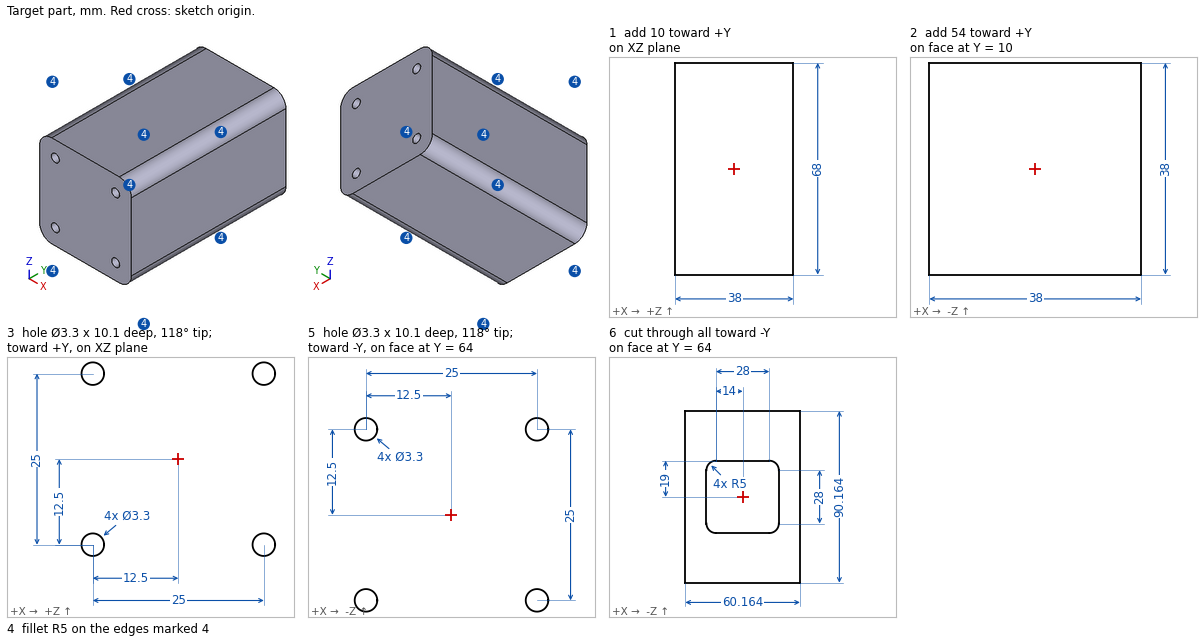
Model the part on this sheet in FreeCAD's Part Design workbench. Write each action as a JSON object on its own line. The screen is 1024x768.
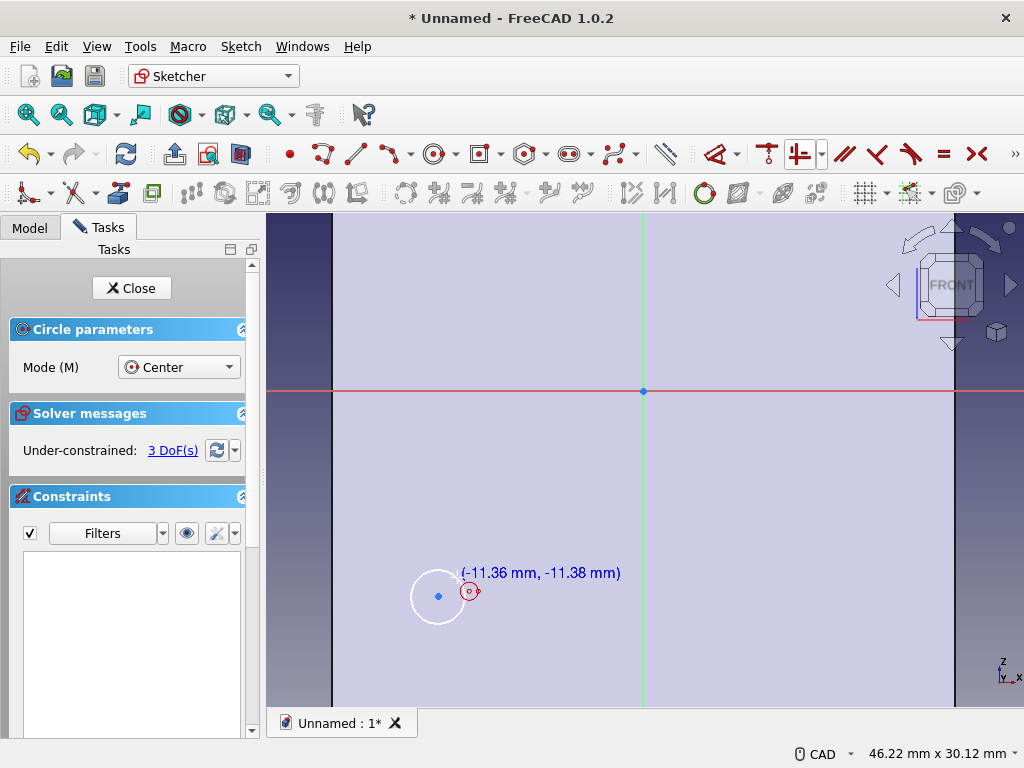
{"action": "left_click", "coordinate": [848, 596]}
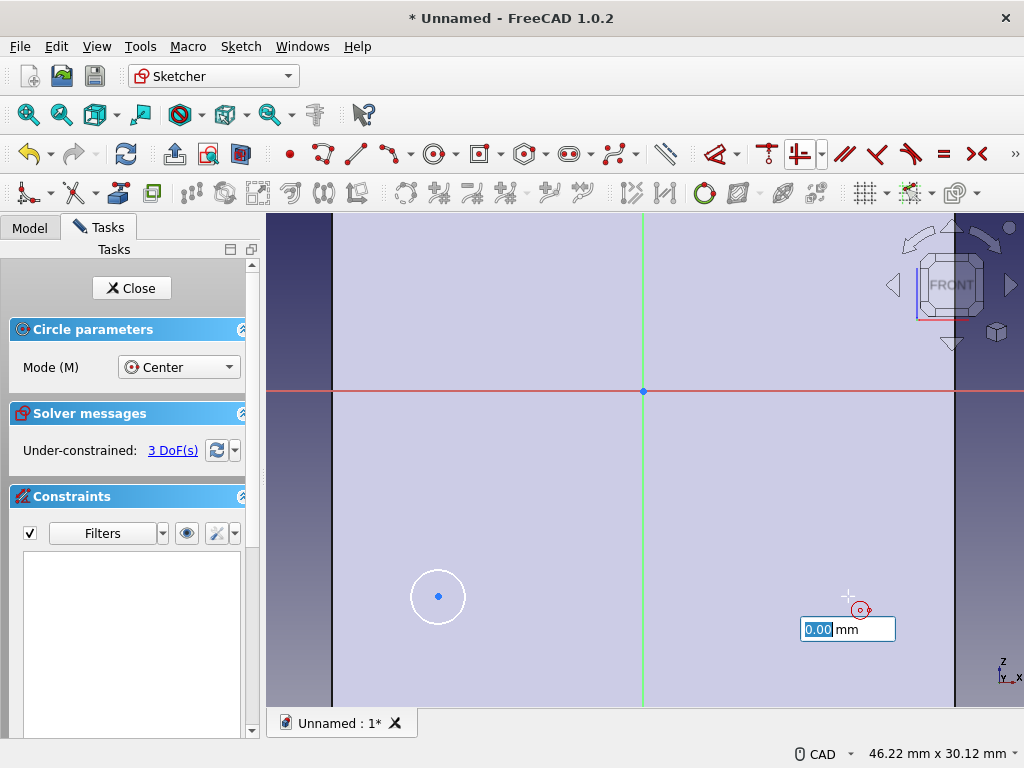
{"action": "scroll", "coordinate": [441, 600], "scroll_direction": "down", "scroll_amount": 2}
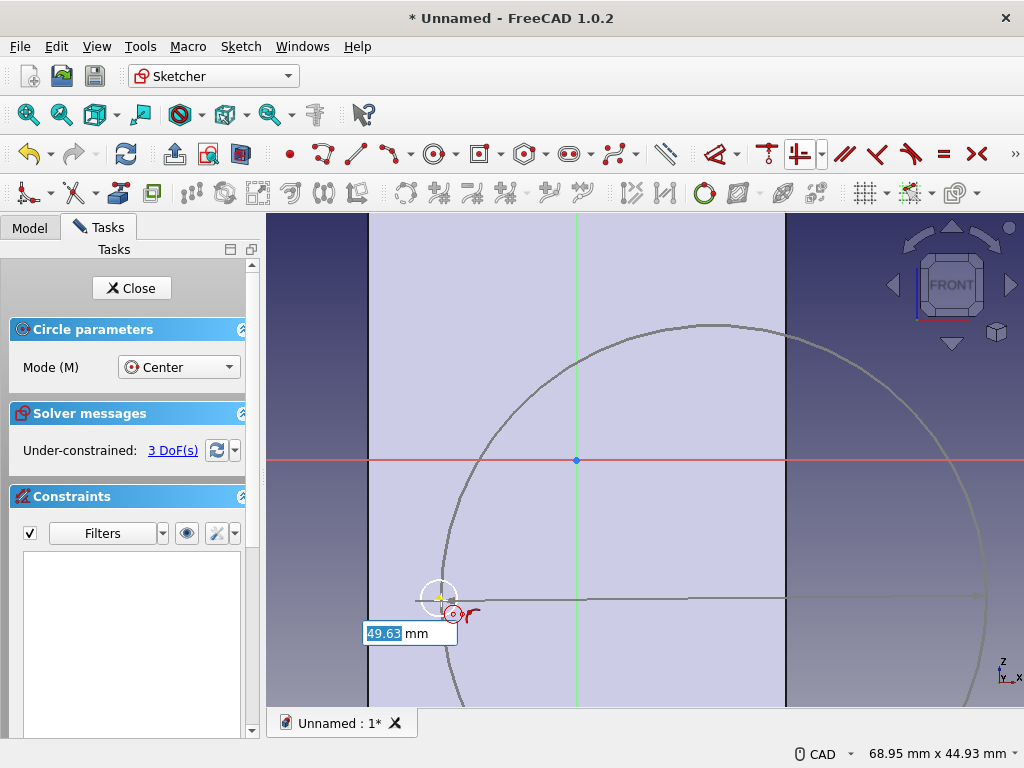
{"action": "left_click", "coordinate": [727, 585]}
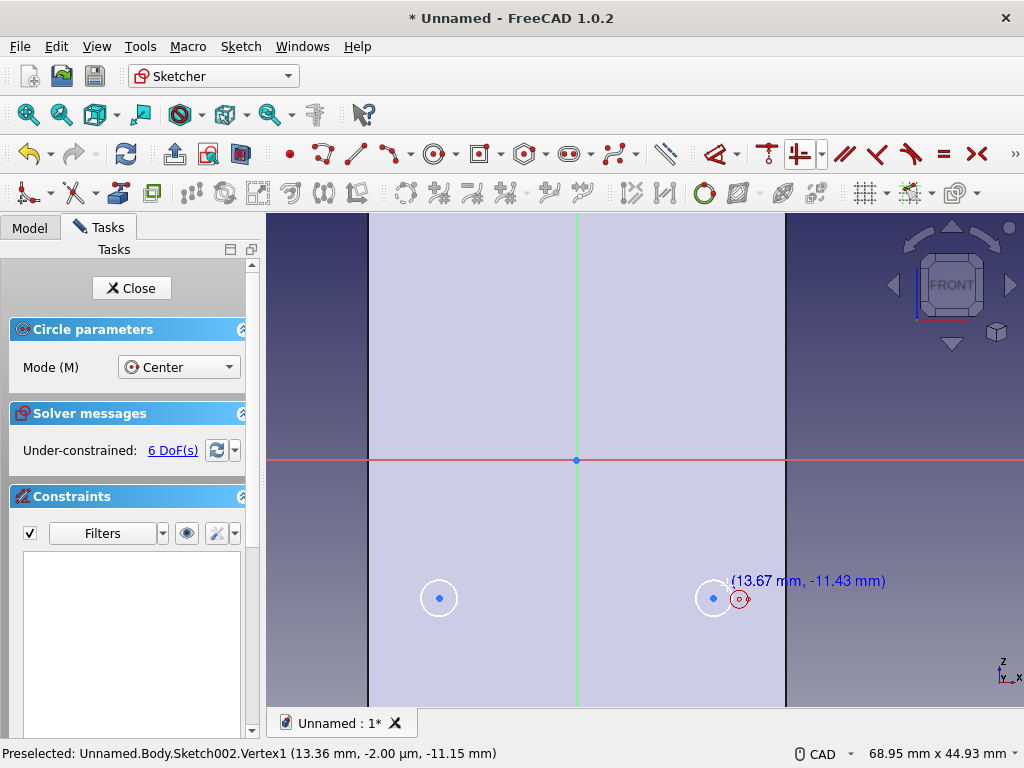
{"action": "scroll", "coordinate": [439, 323], "scroll_direction": "up", "scroll_amount": 2}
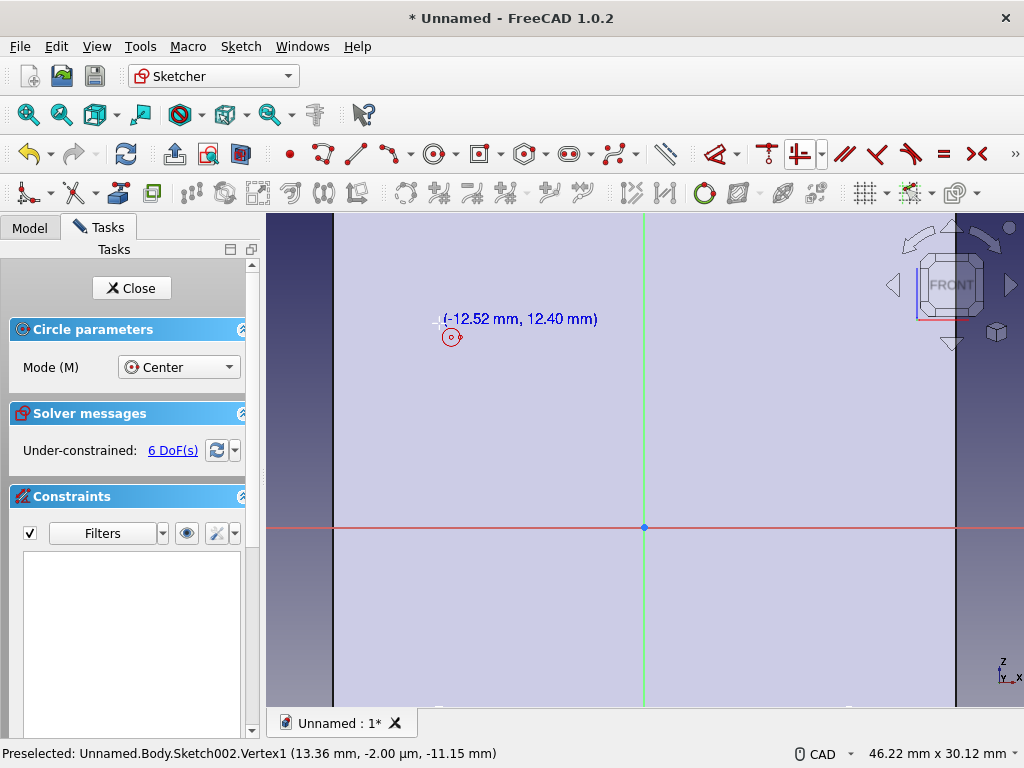
{"action": "left_click", "coordinate": [439, 323]}
{"action": "left_click", "coordinate": [458, 304]}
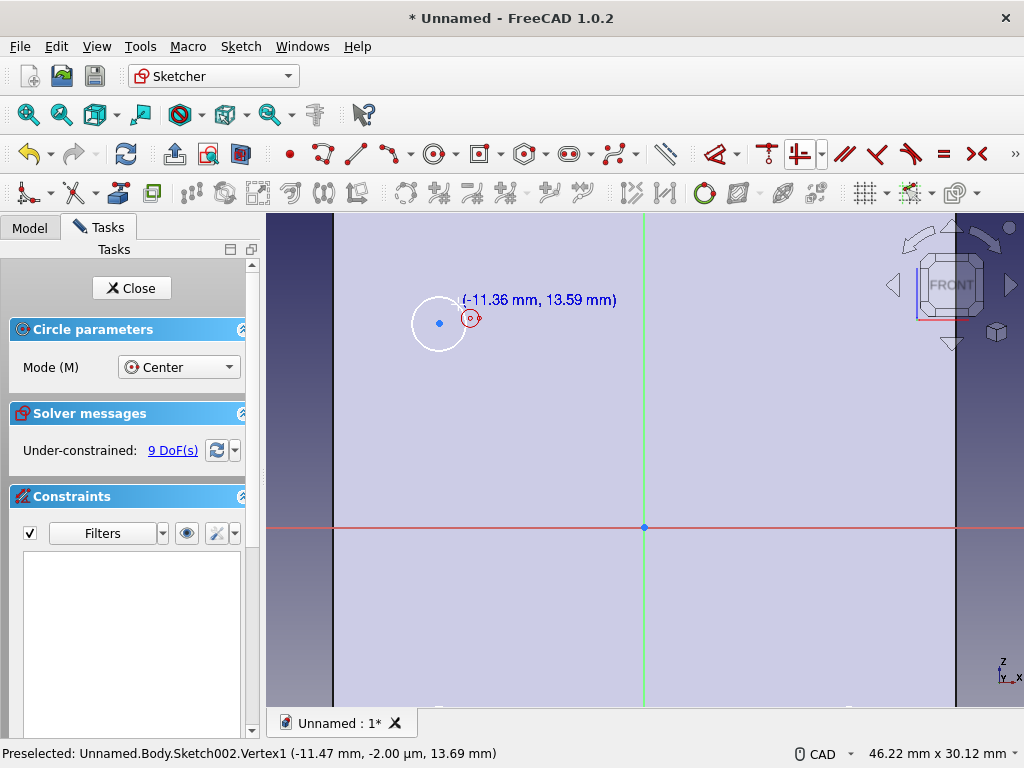
{"action": "left_click", "coordinate": [849, 323]}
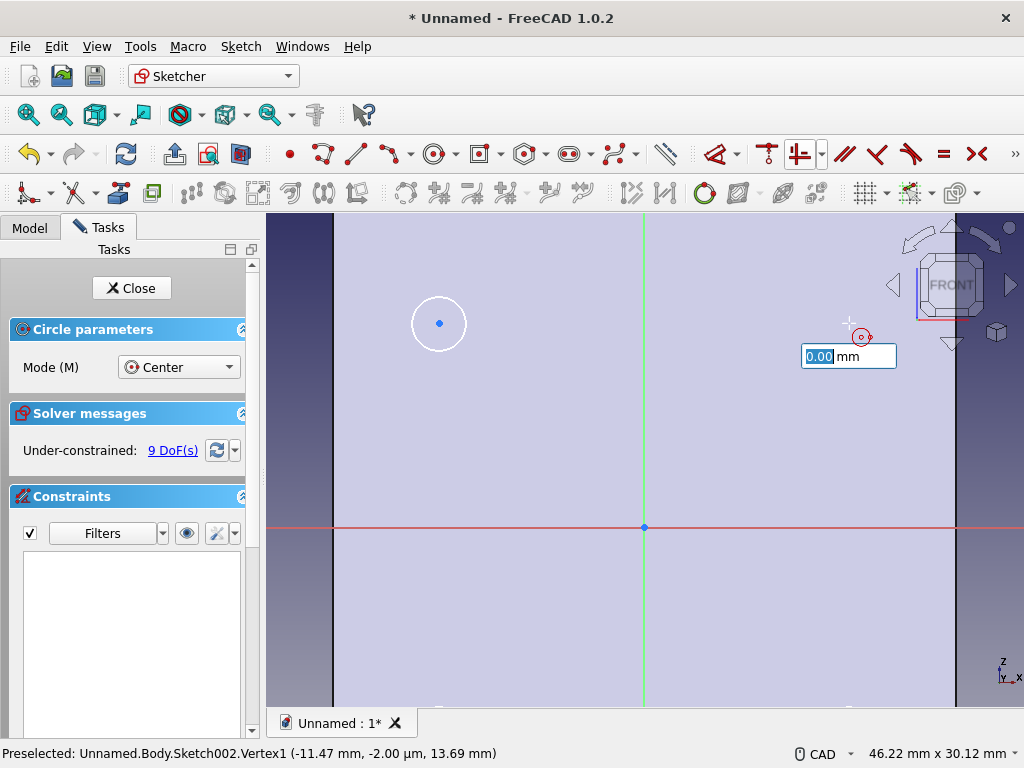
{"action": "scroll", "coordinate": [439, 322], "scroll_direction": "down", "scroll_amount": 2}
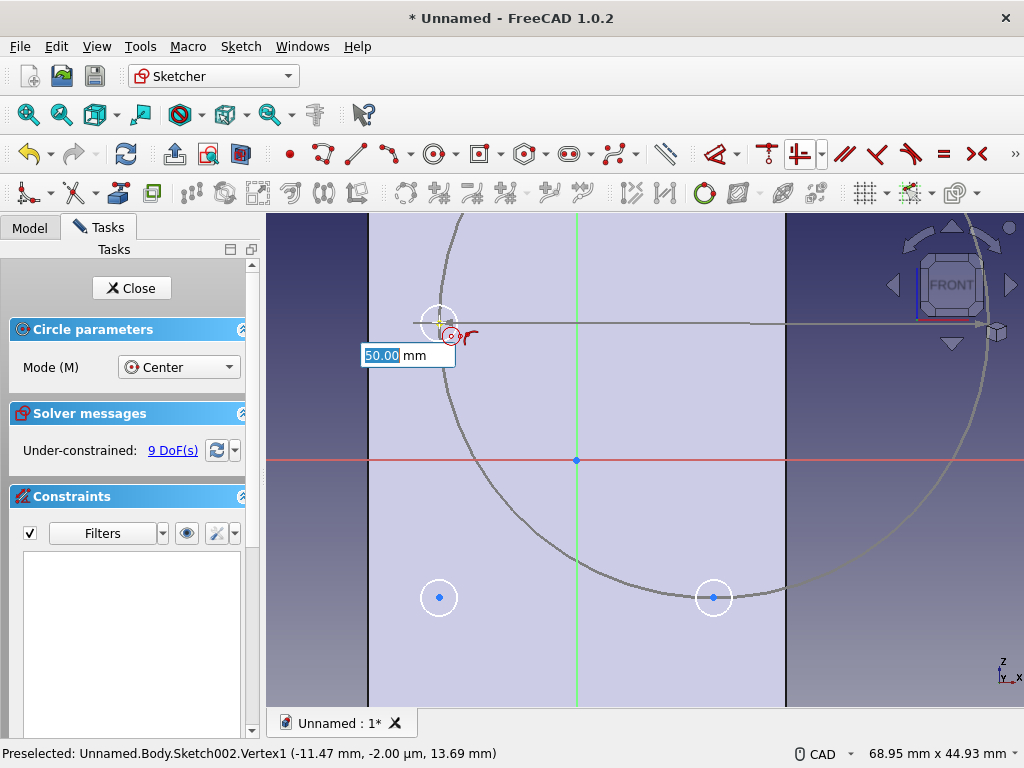
{"action": "left_click", "coordinate": [727, 310]}
{"action": "key", "text": "Escape"}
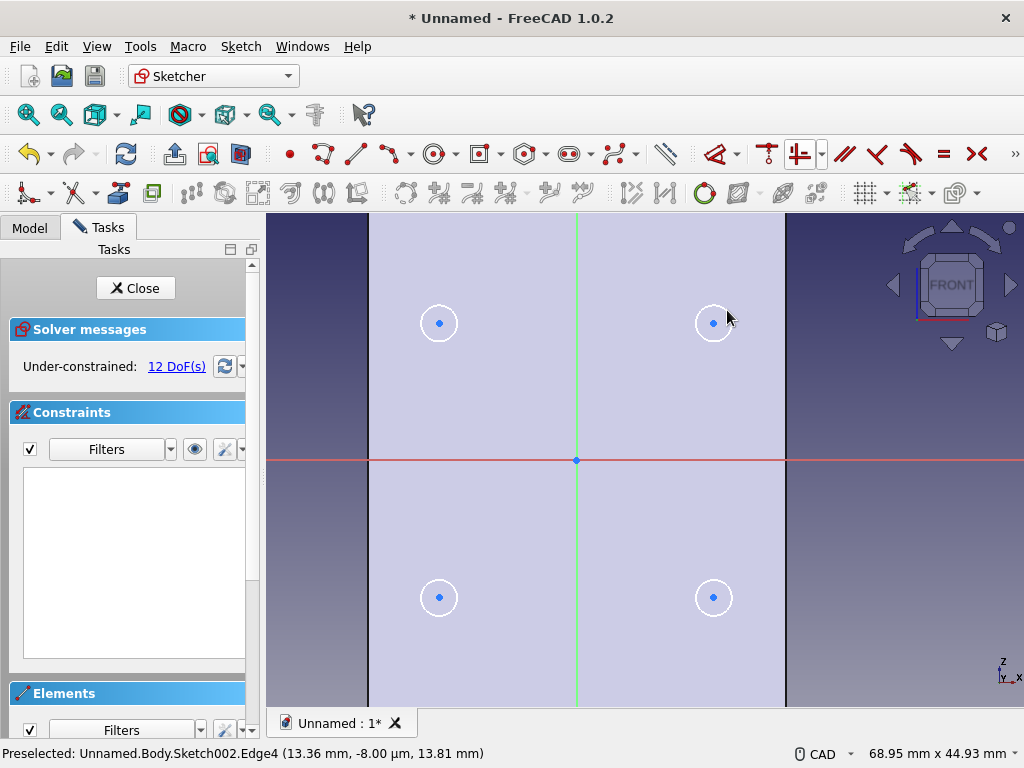
{"action": "left_click", "coordinate": [452, 585]}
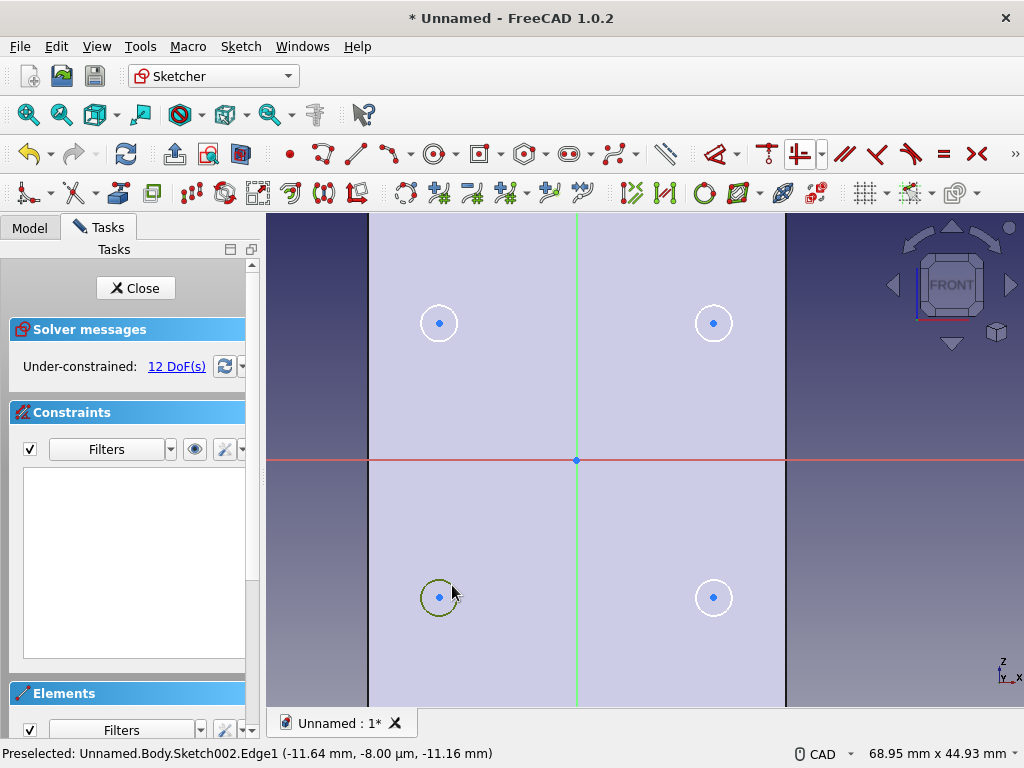
{"action": "left_click", "coordinate": [727, 585]}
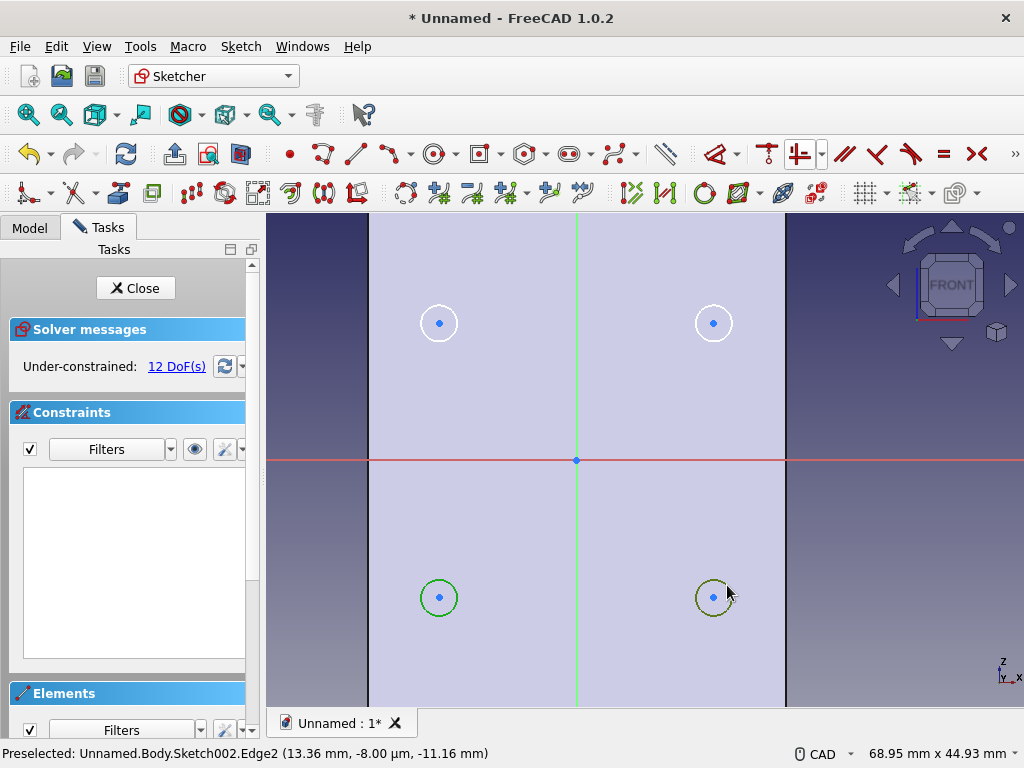
{"action": "left_click", "coordinate": [452, 311]}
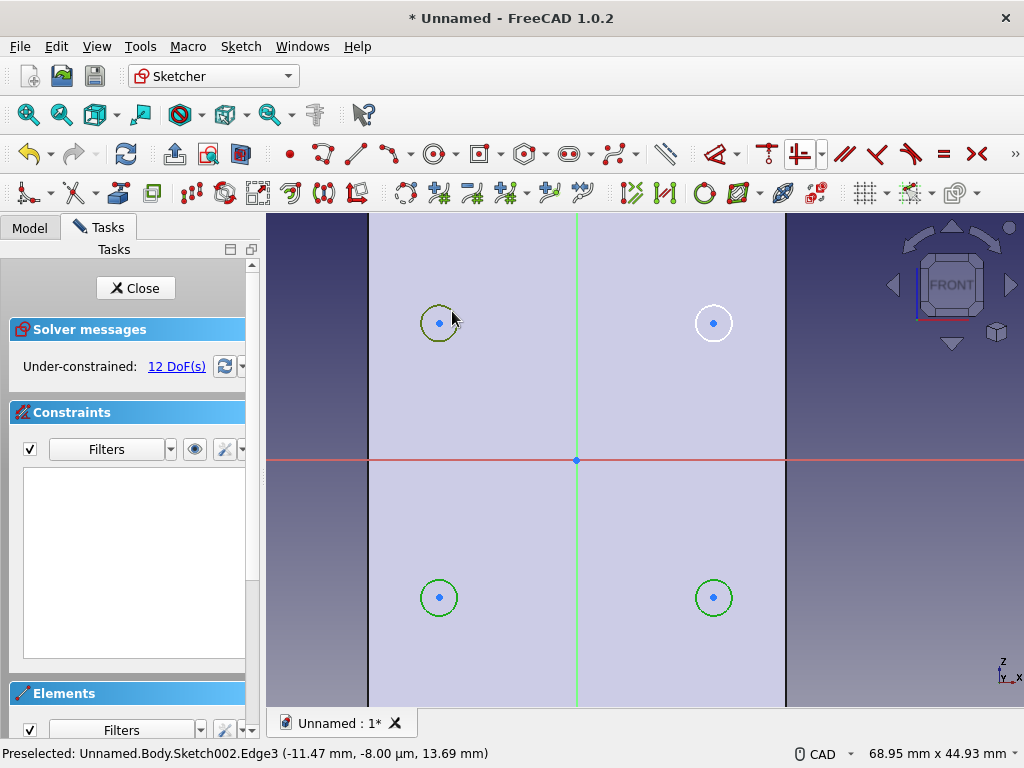
{"action": "left_click", "coordinate": [727, 311]}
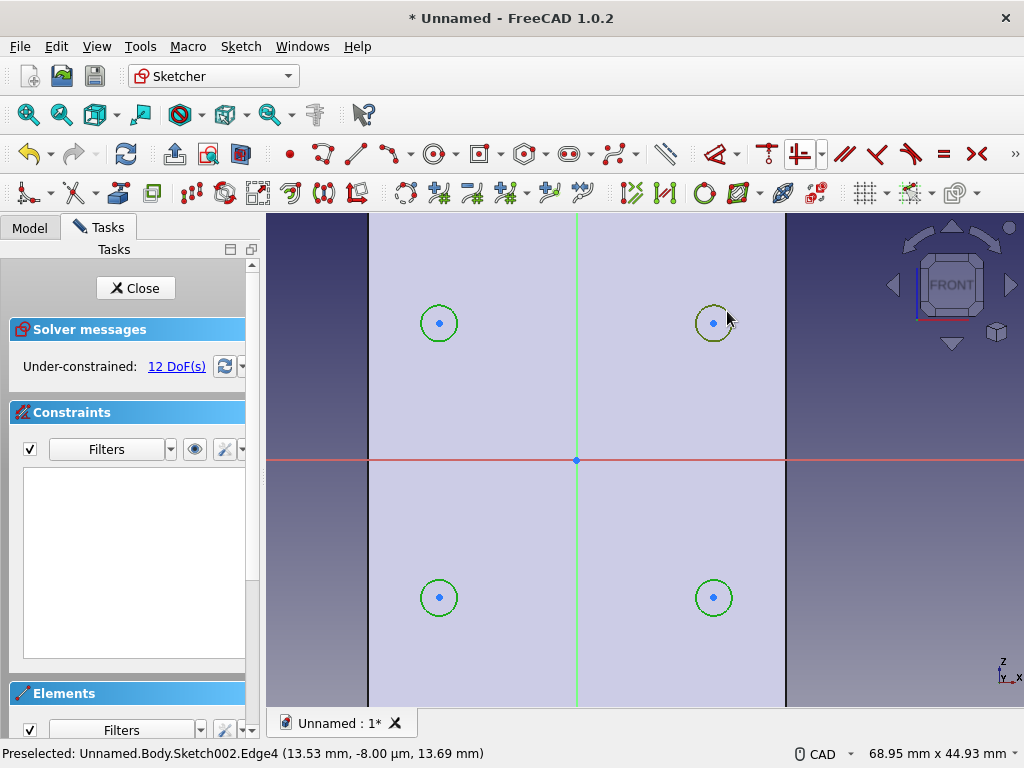
{"action": "key", "text": "e"}